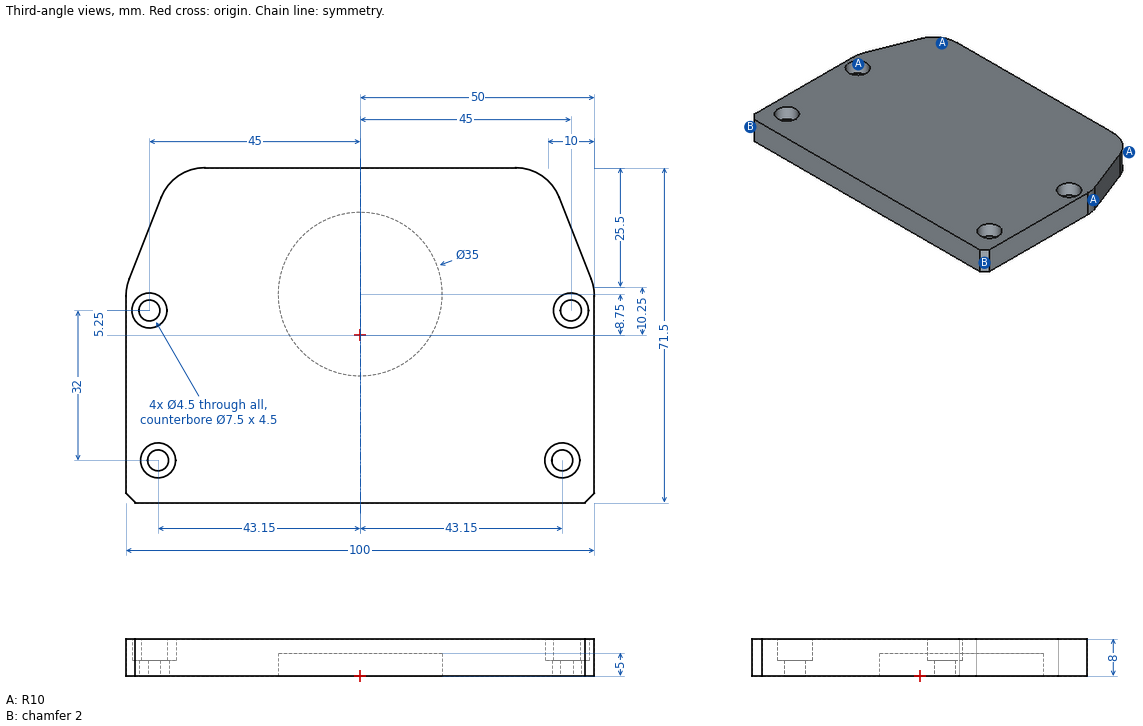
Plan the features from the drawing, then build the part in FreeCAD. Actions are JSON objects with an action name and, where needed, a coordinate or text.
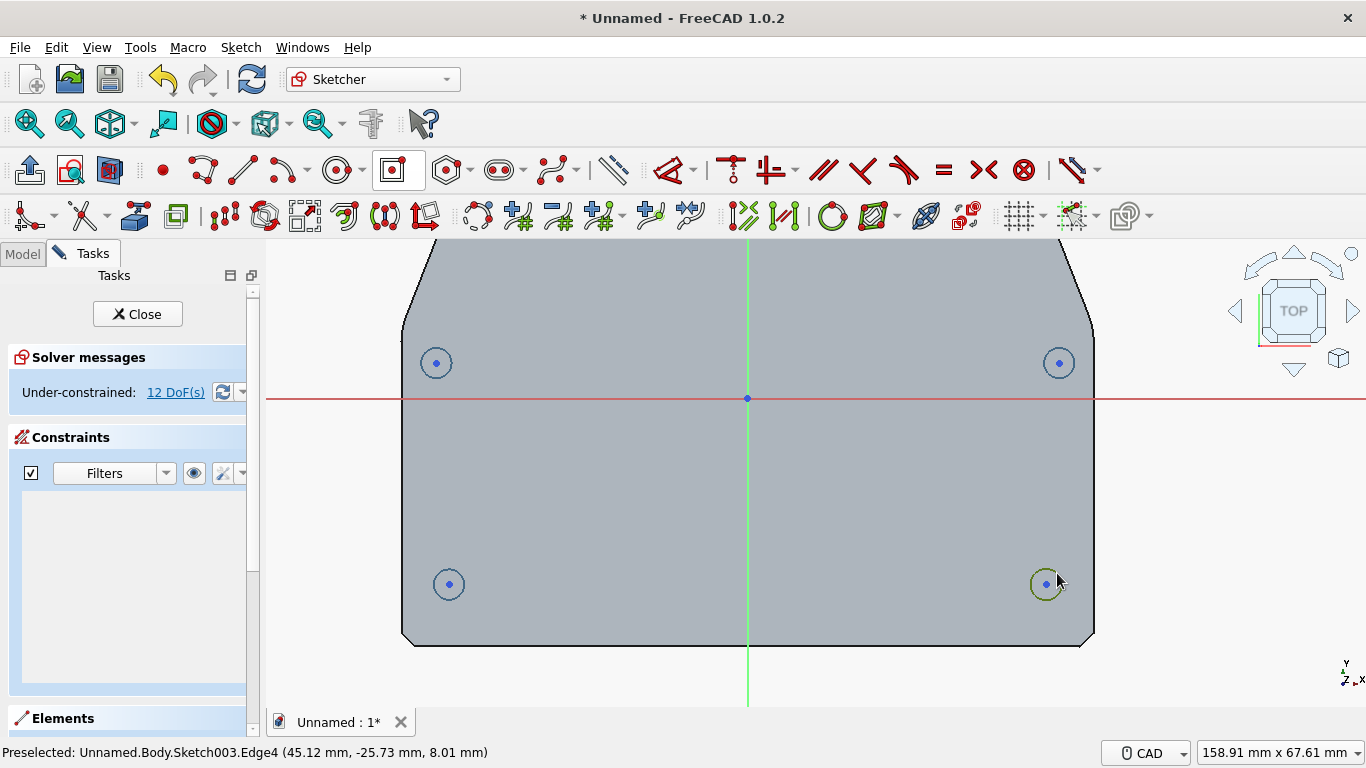
{"action": "left_click", "coordinate": [944, 170]}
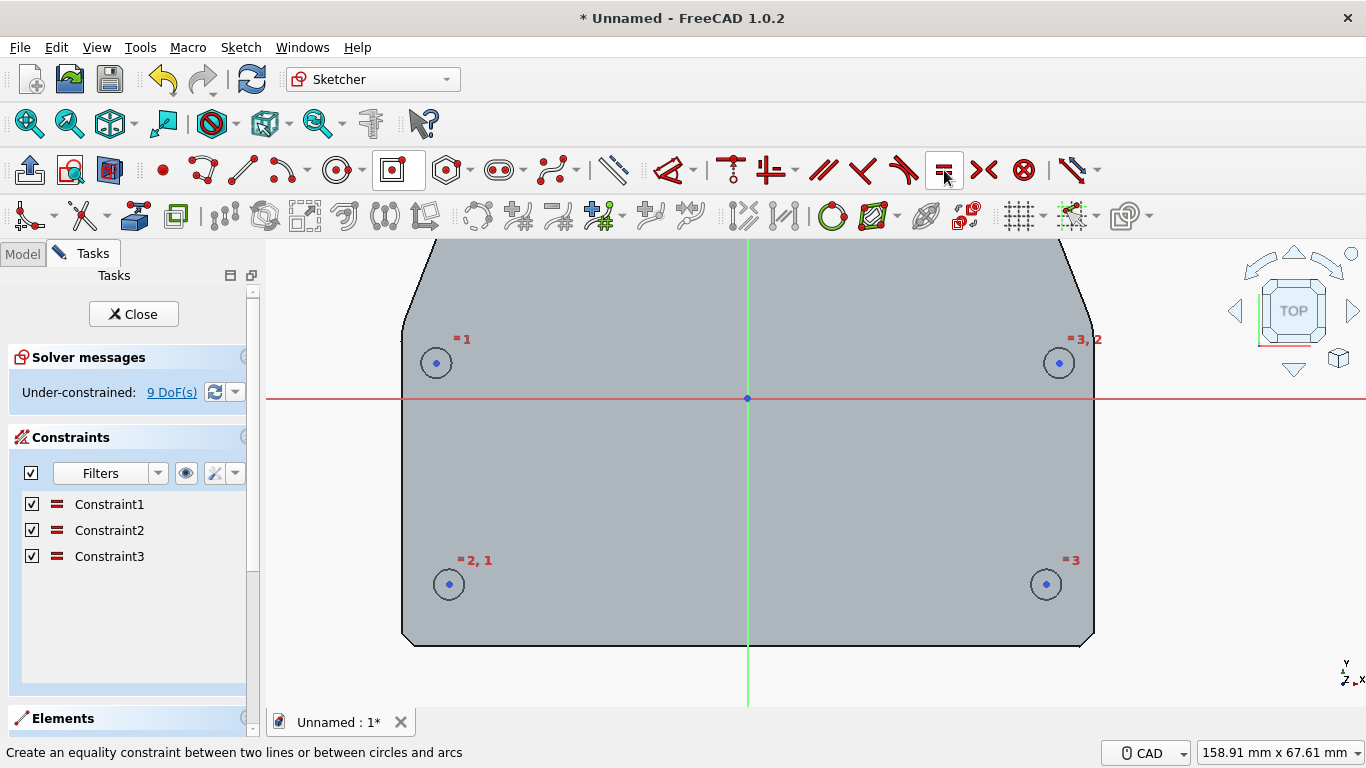
{"action": "left_click", "coordinate": [436, 363]}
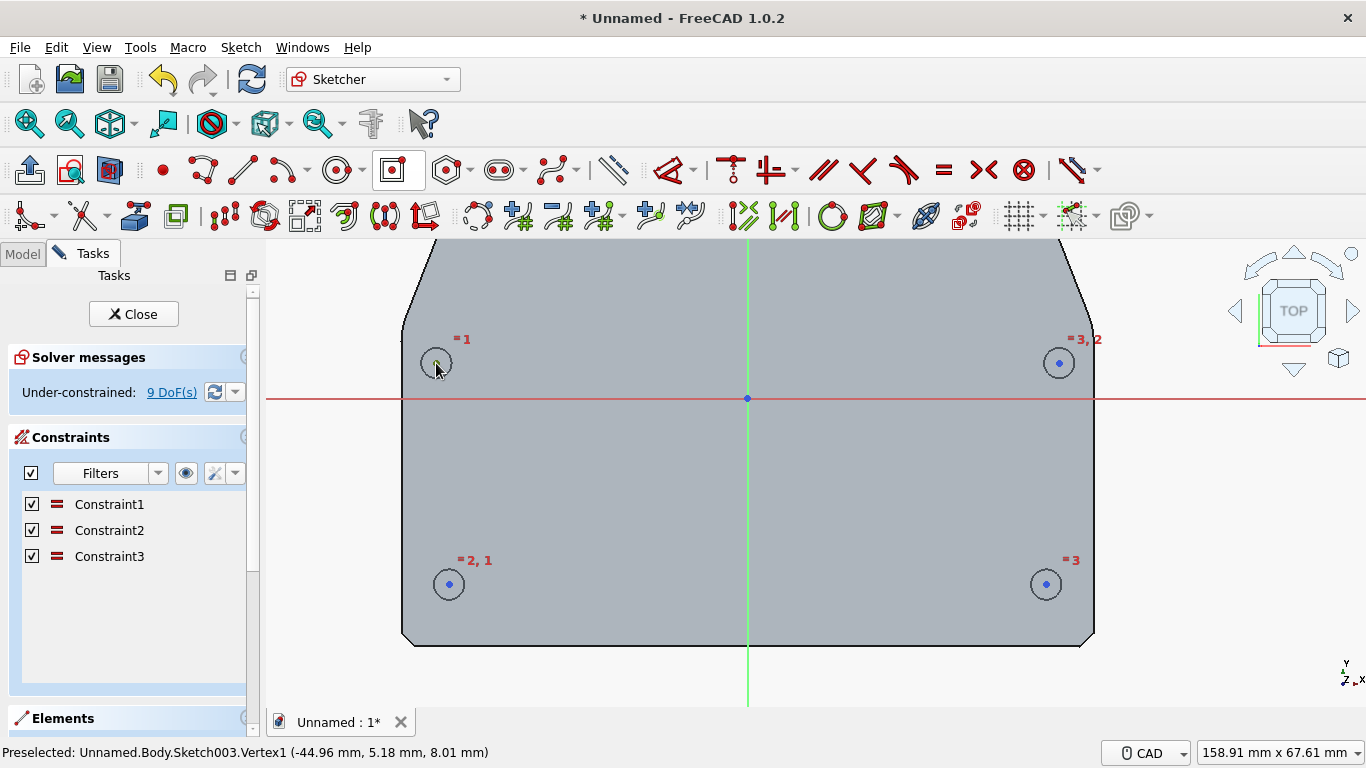
{"action": "left_click", "coordinate": [1059, 363]}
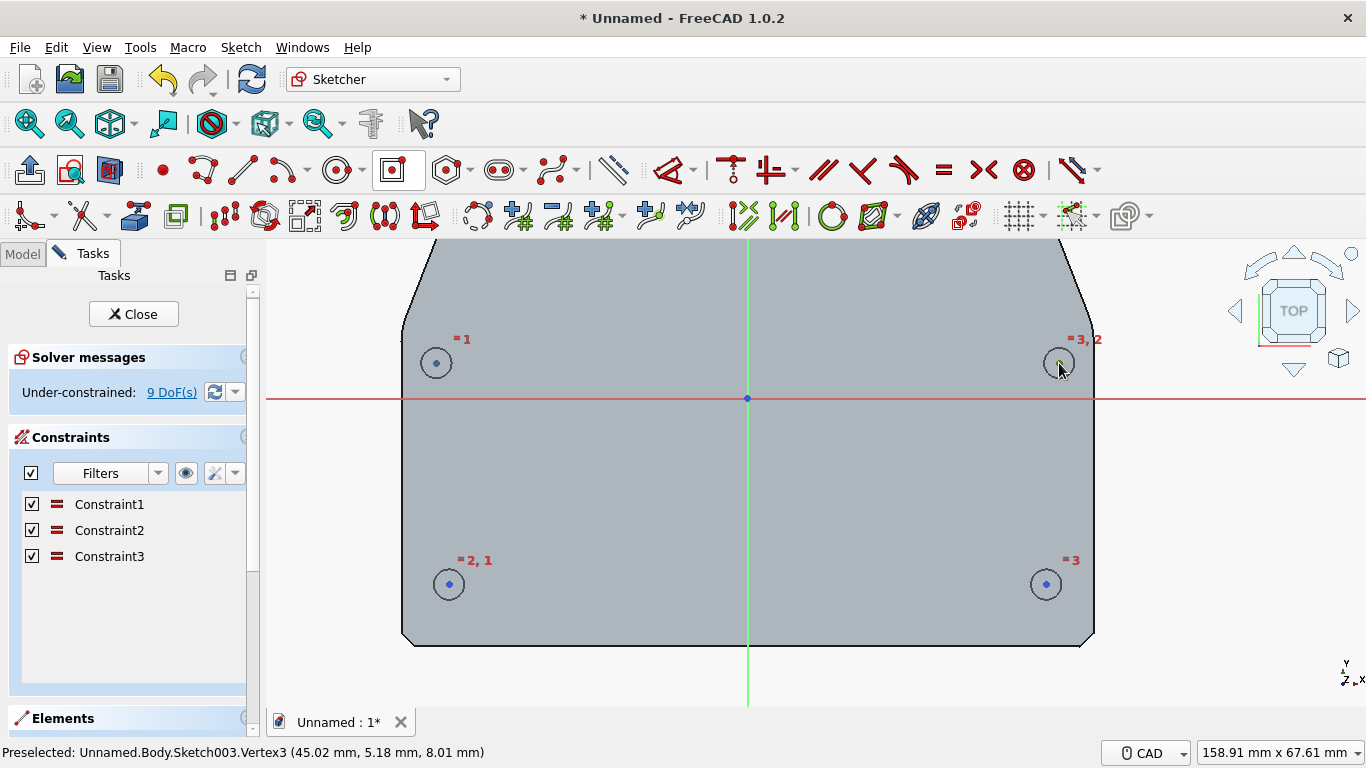
{"action": "left_click", "coordinate": [798, 170]}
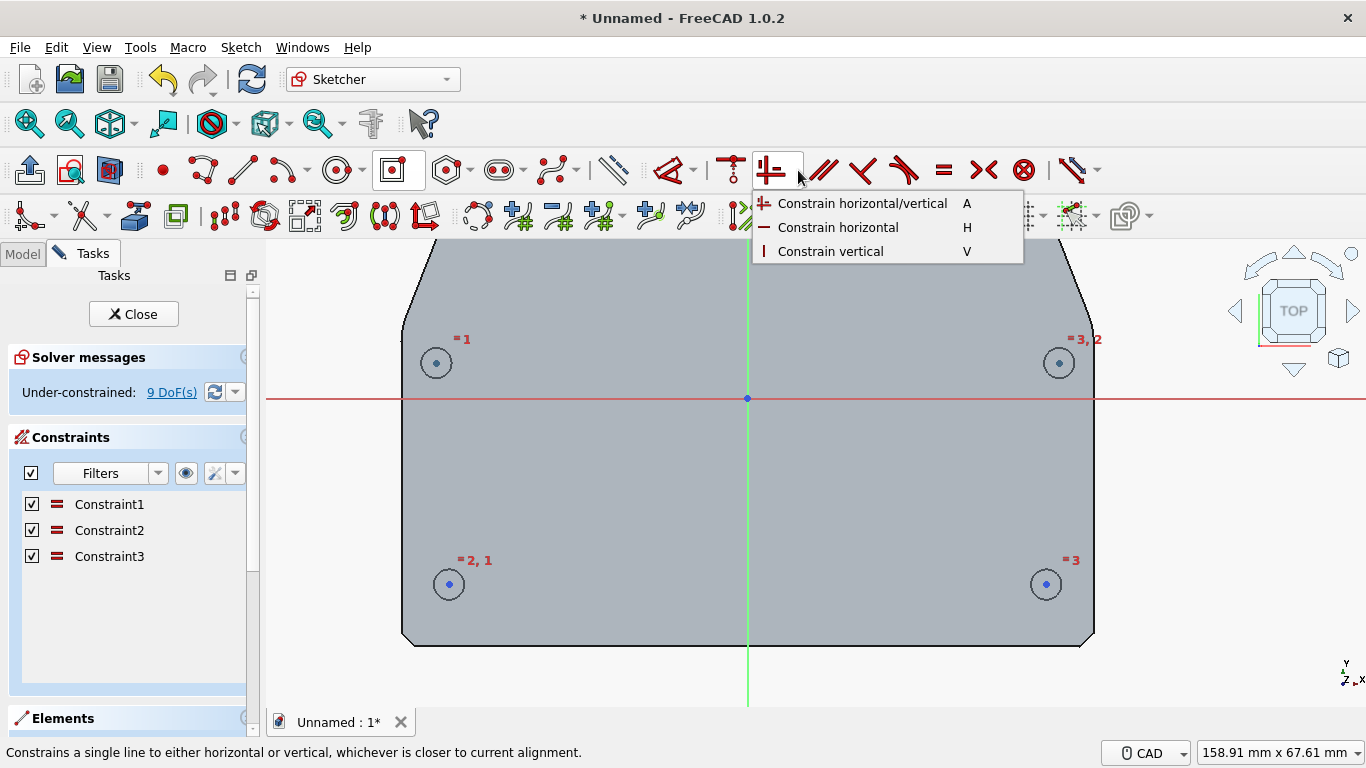
{"action": "left_click", "coordinate": [888, 227]}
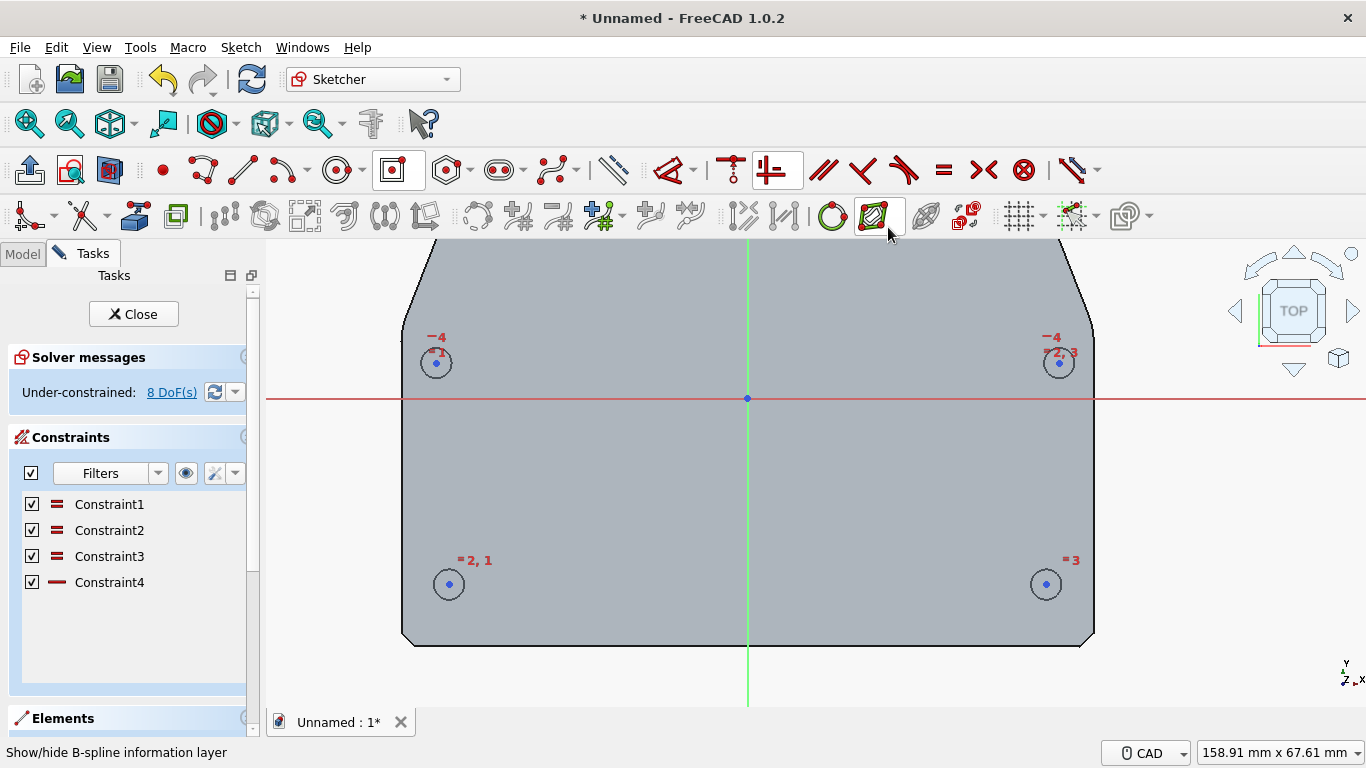
{"action": "left_click", "coordinate": [449, 585]}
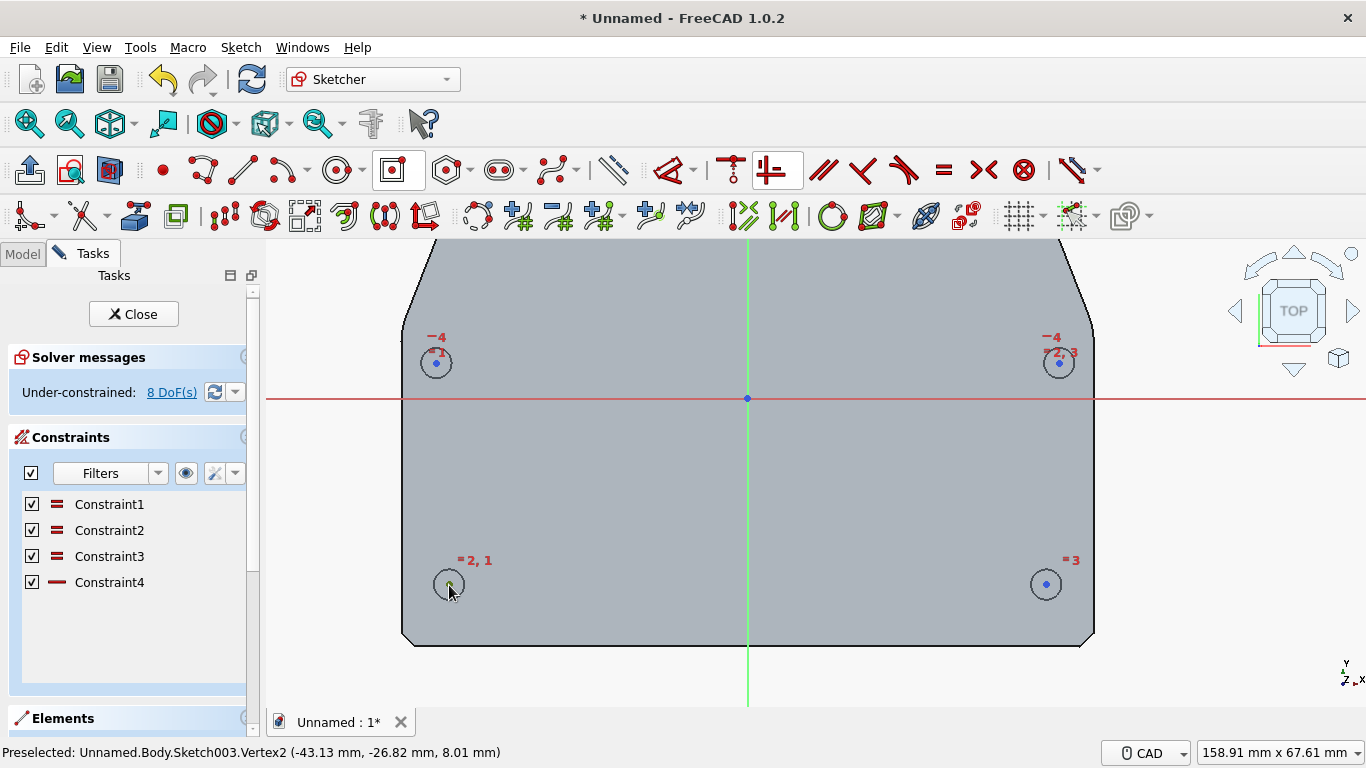
{"action": "left_click", "coordinate": [1046, 585]}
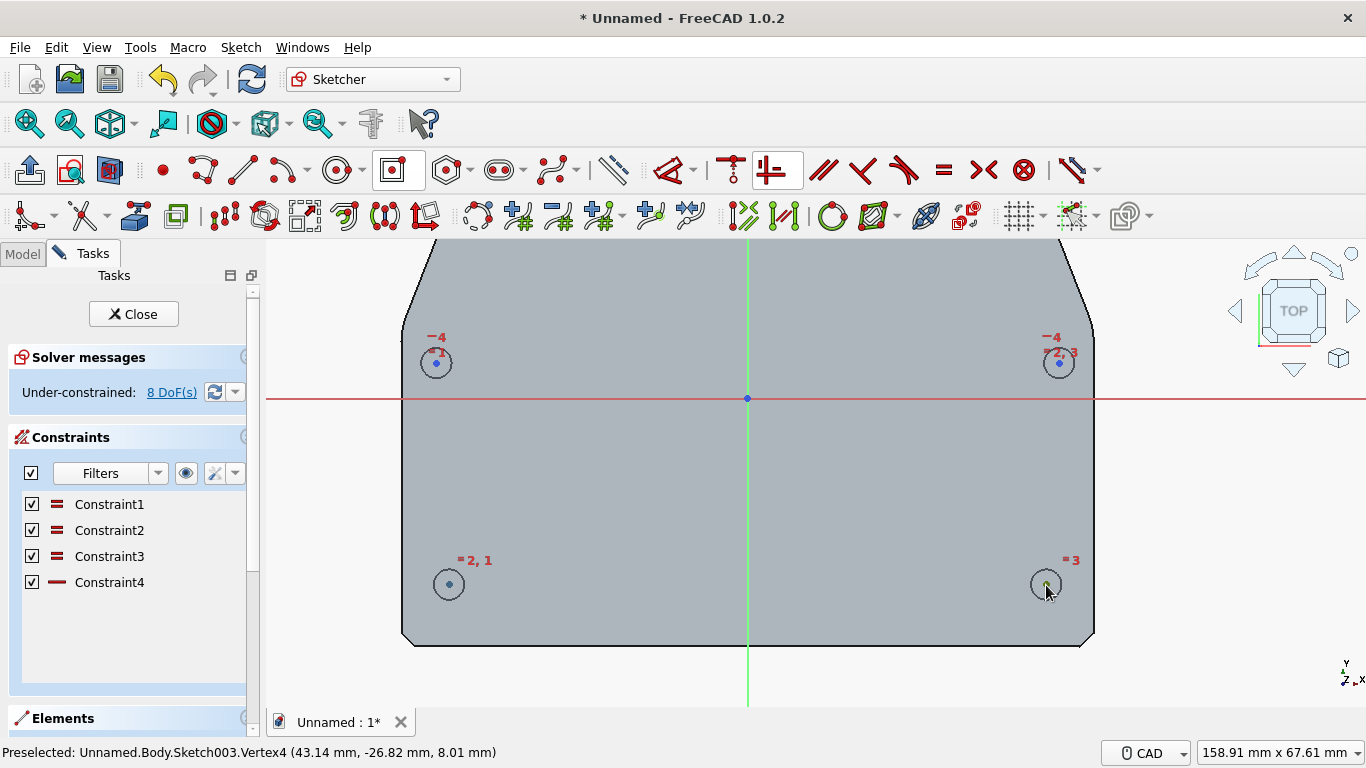
{"action": "left_click", "coordinate": [798, 170]}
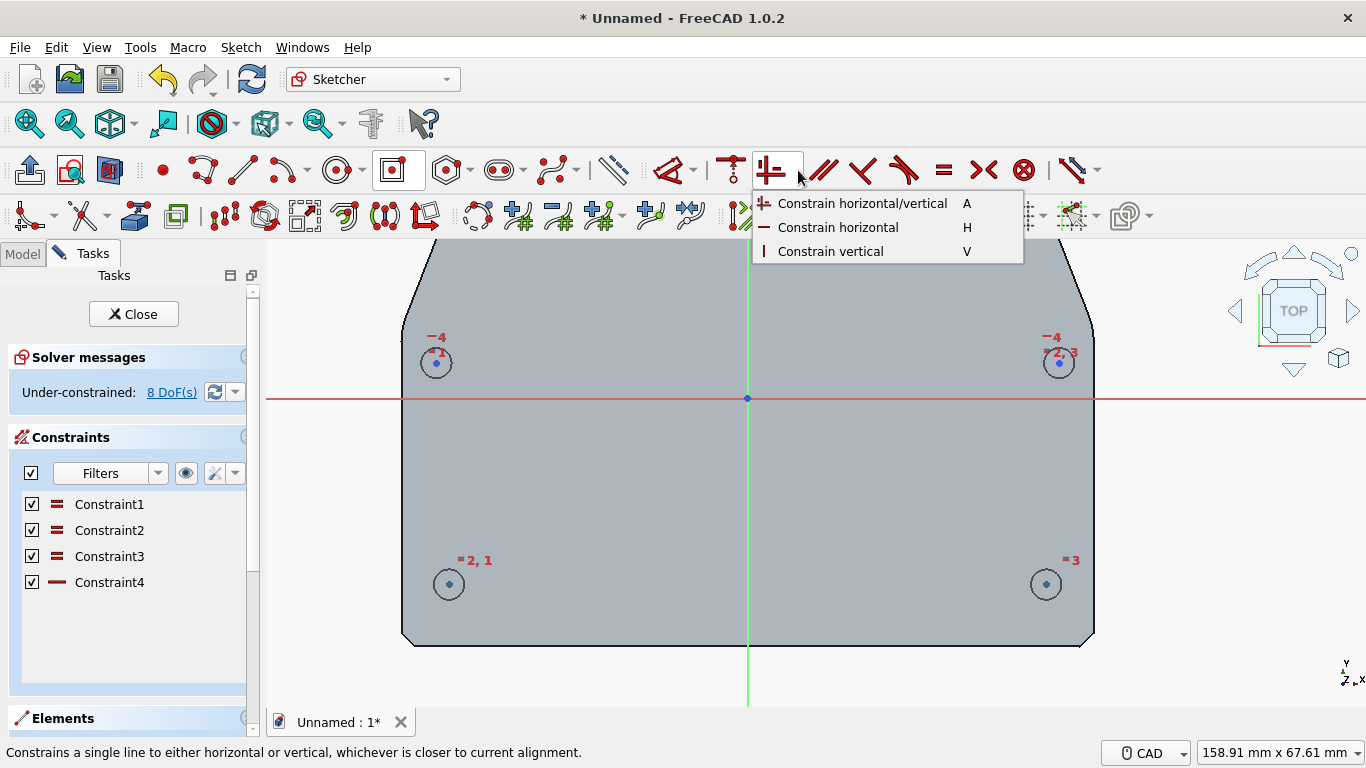
{"action": "left_click", "coordinate": [888, 227]}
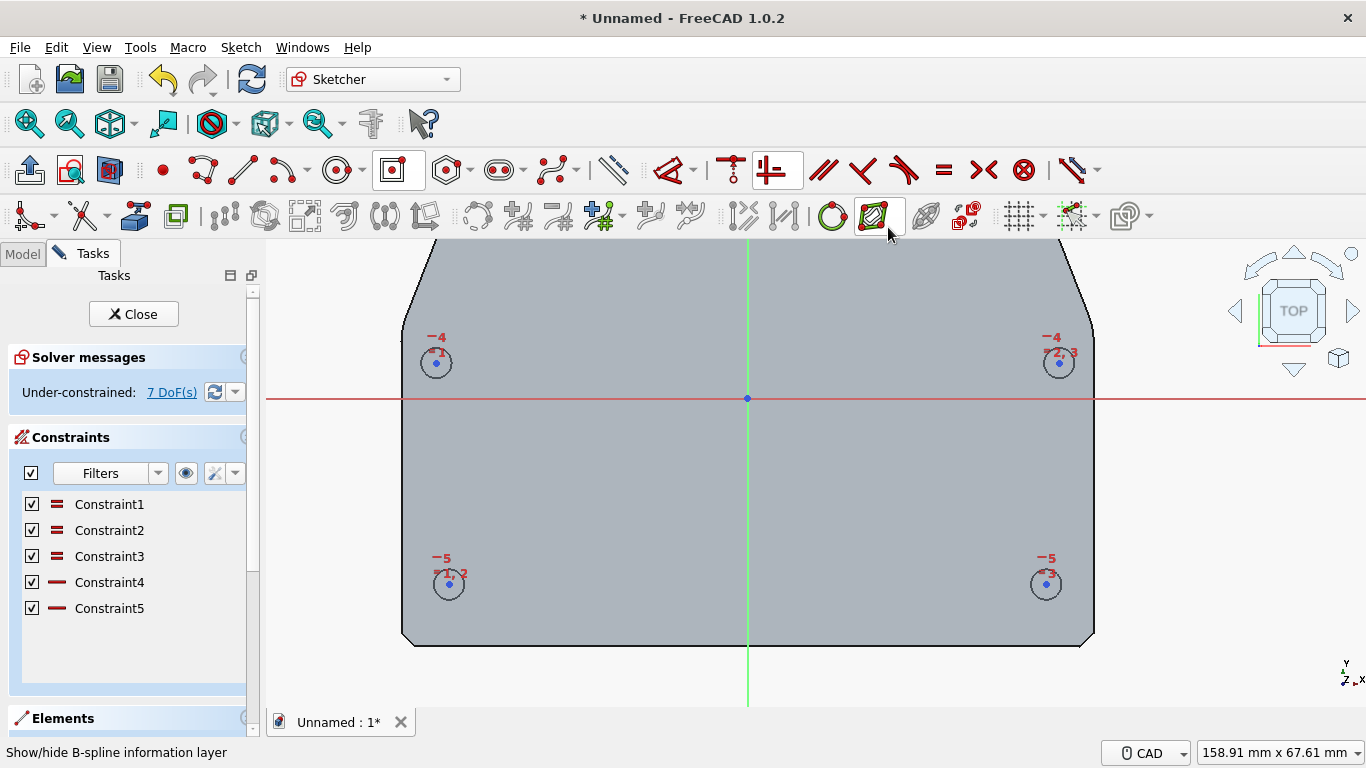
{"action": "left_click", "coordinate": [668, 170]}